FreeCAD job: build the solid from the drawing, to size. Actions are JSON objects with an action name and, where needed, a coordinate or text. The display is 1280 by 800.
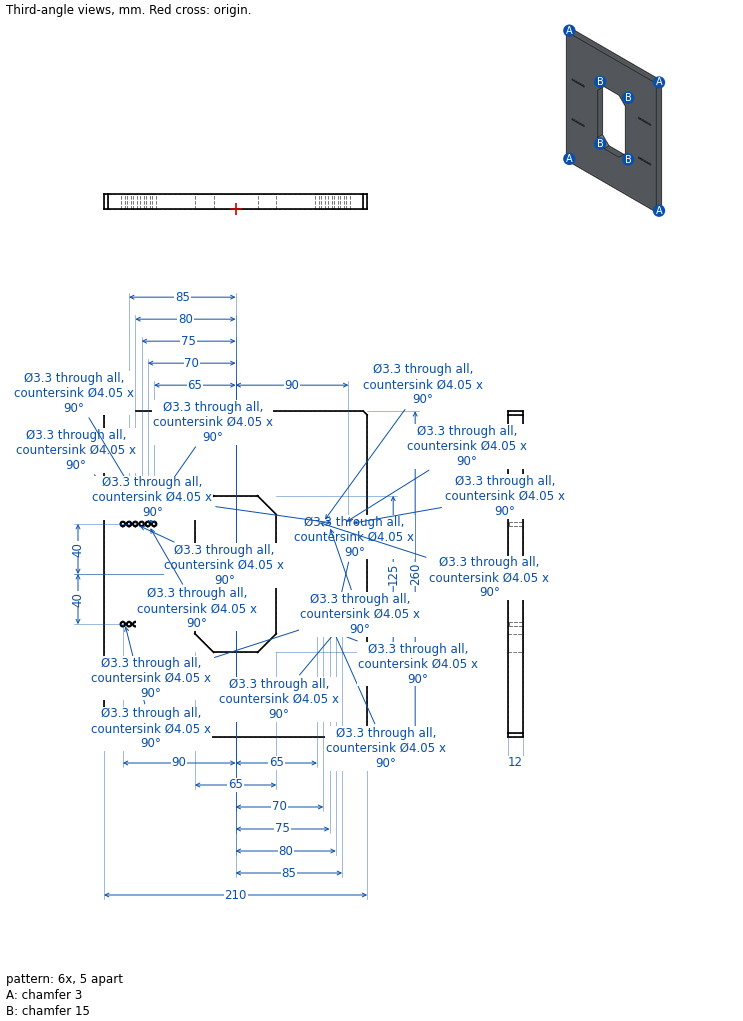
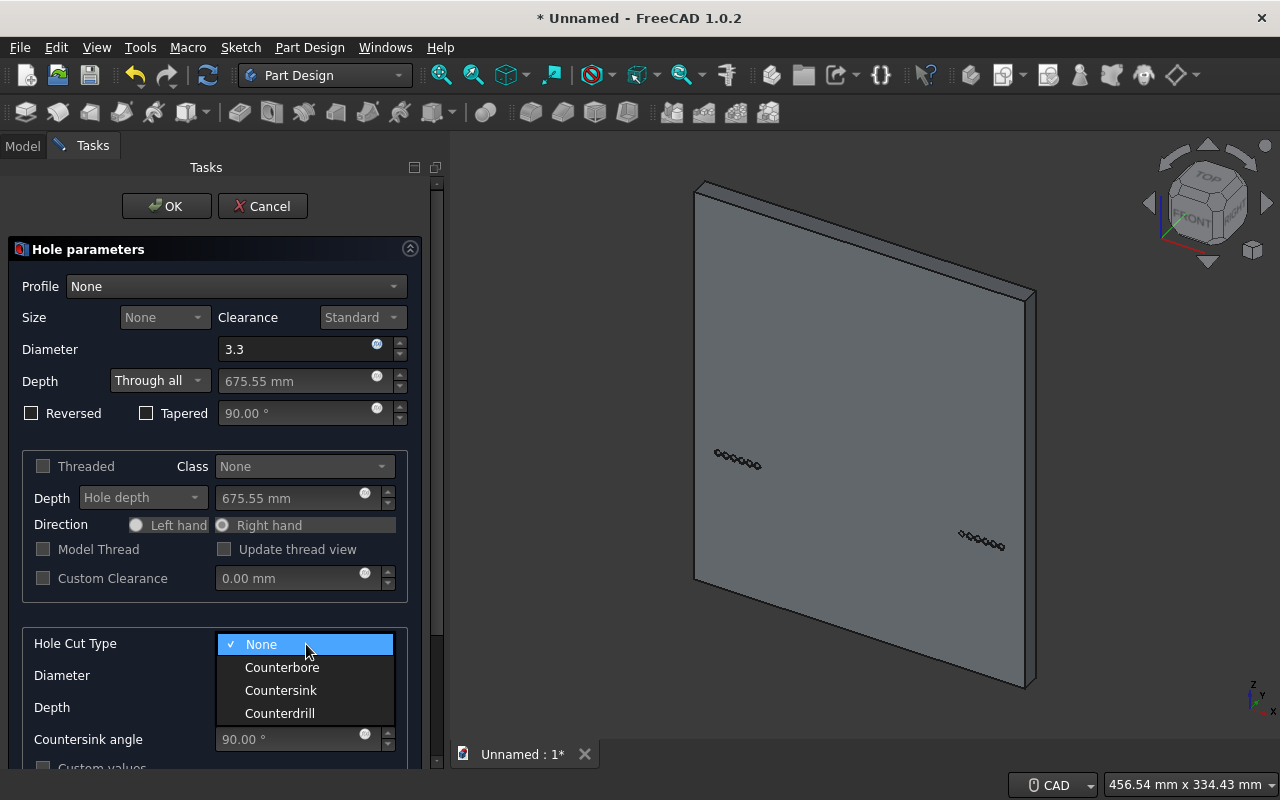
{"action": "left_click", "coordinate": [304, 690]}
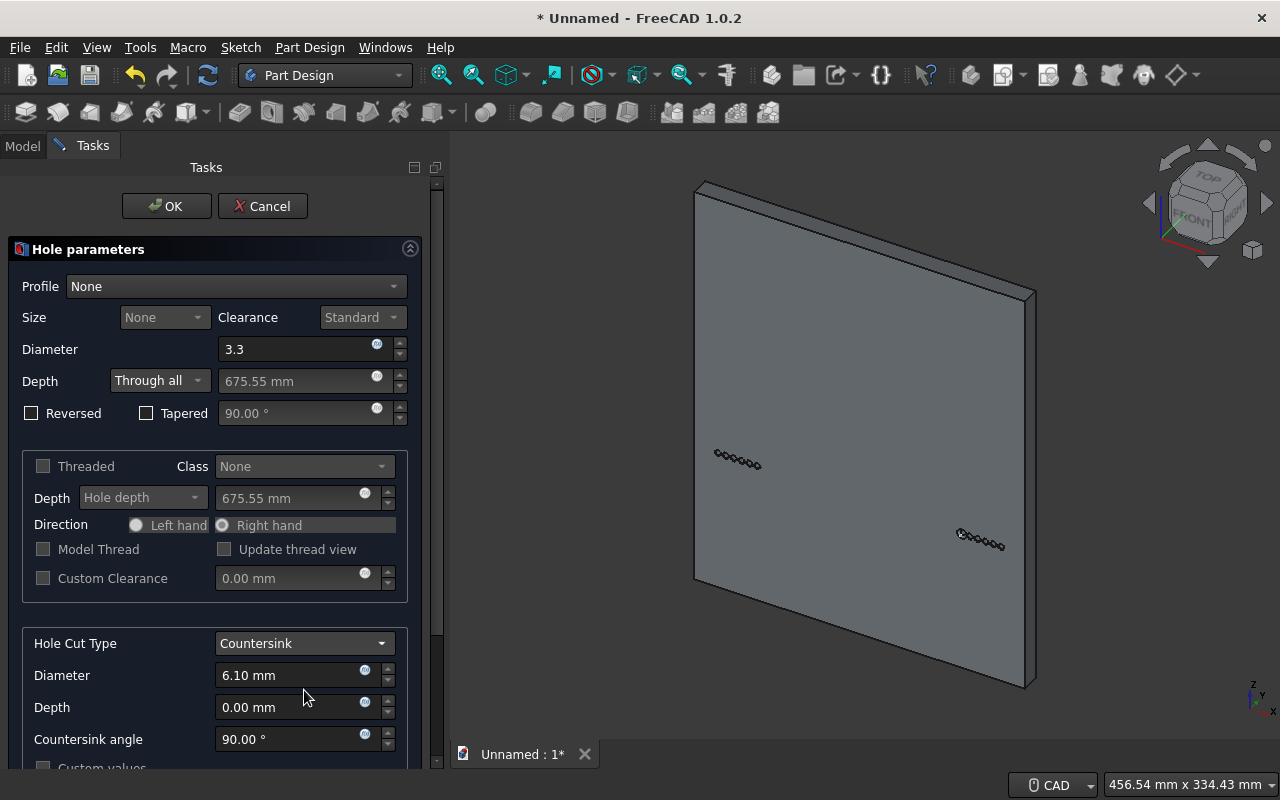
{"action": "triple_click", "coordinate": [298, 675]}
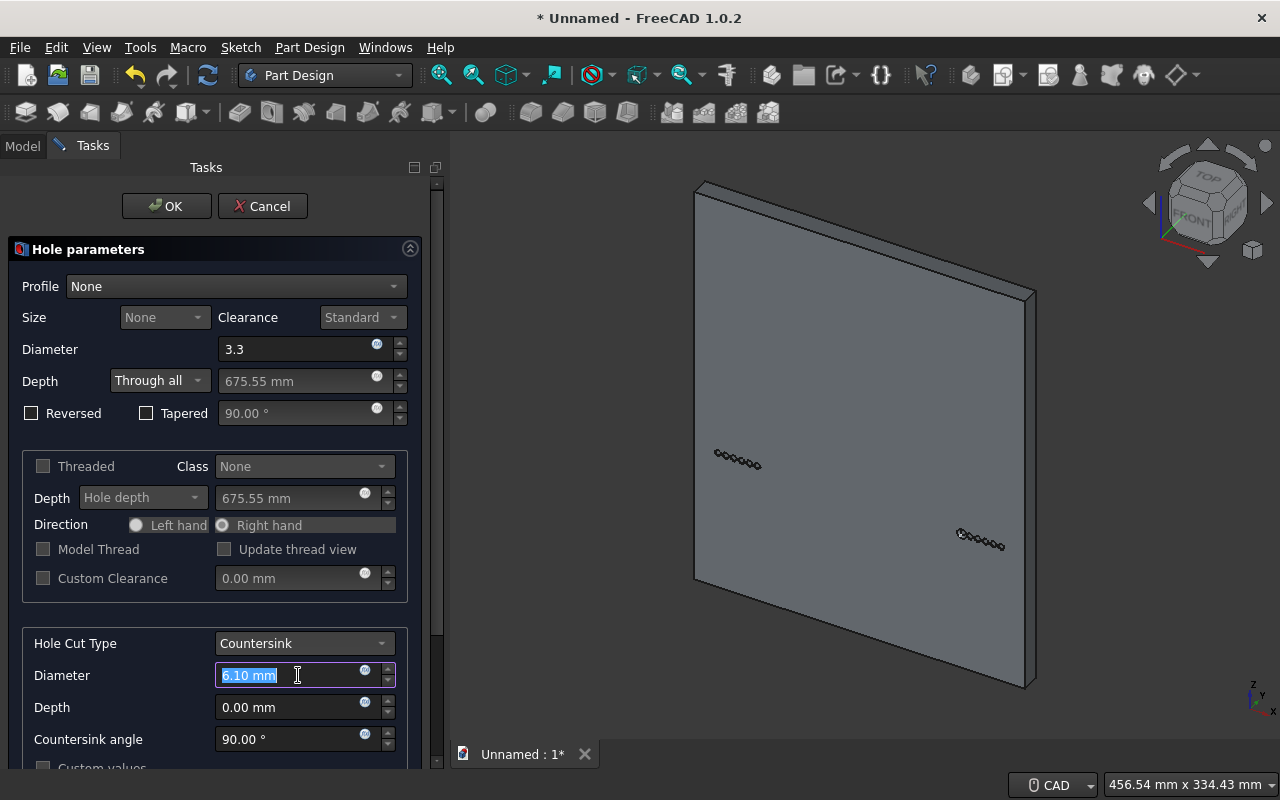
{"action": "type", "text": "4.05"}
{"action": "key", "text": "Tab"}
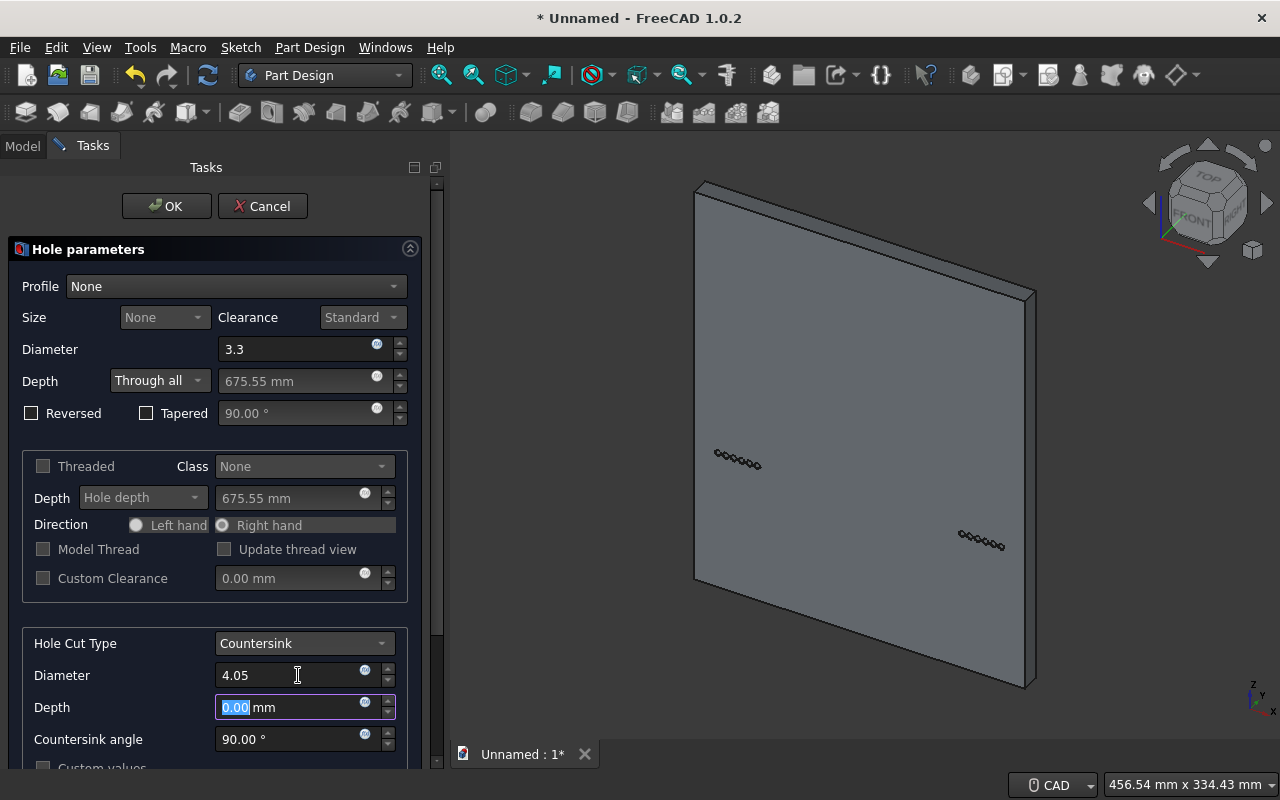
{"action": "left_click", "coordinate": [167, 206]}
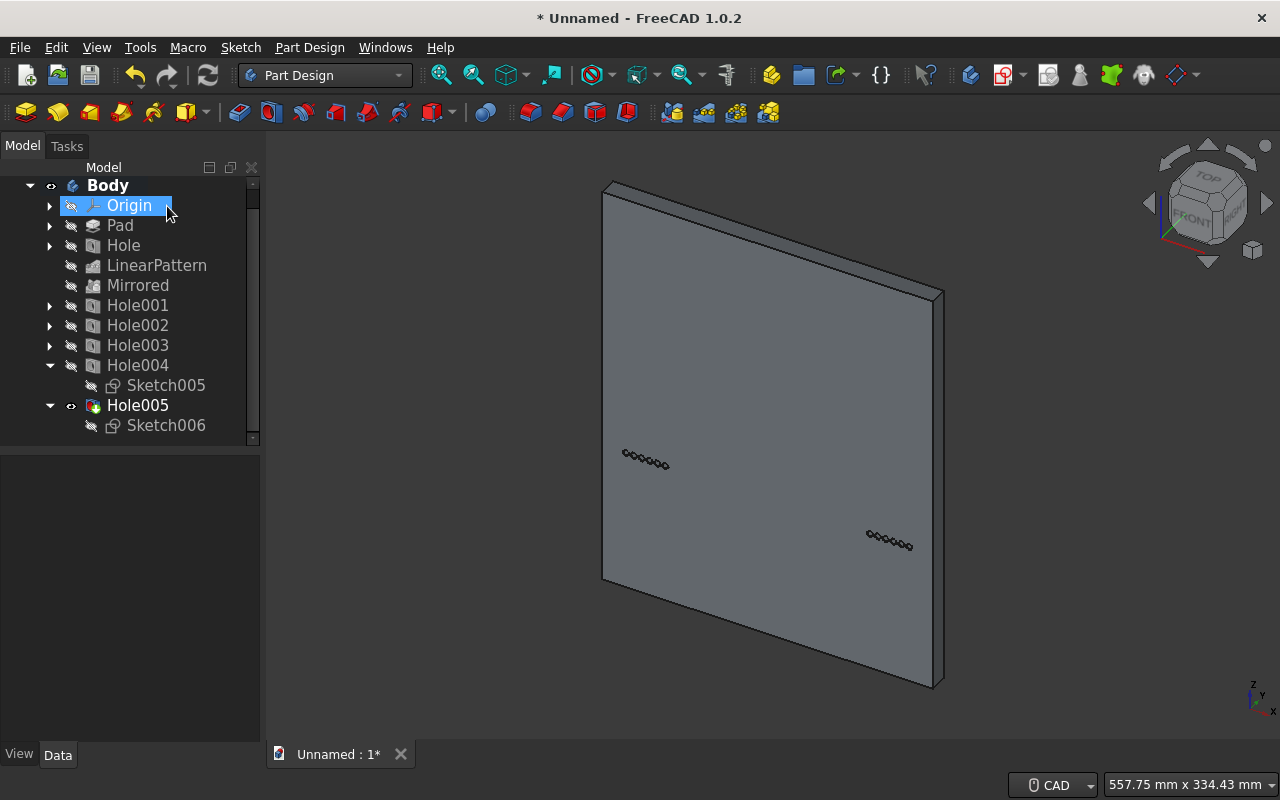
{"action": "left_click", "coordinate": [116, 246]}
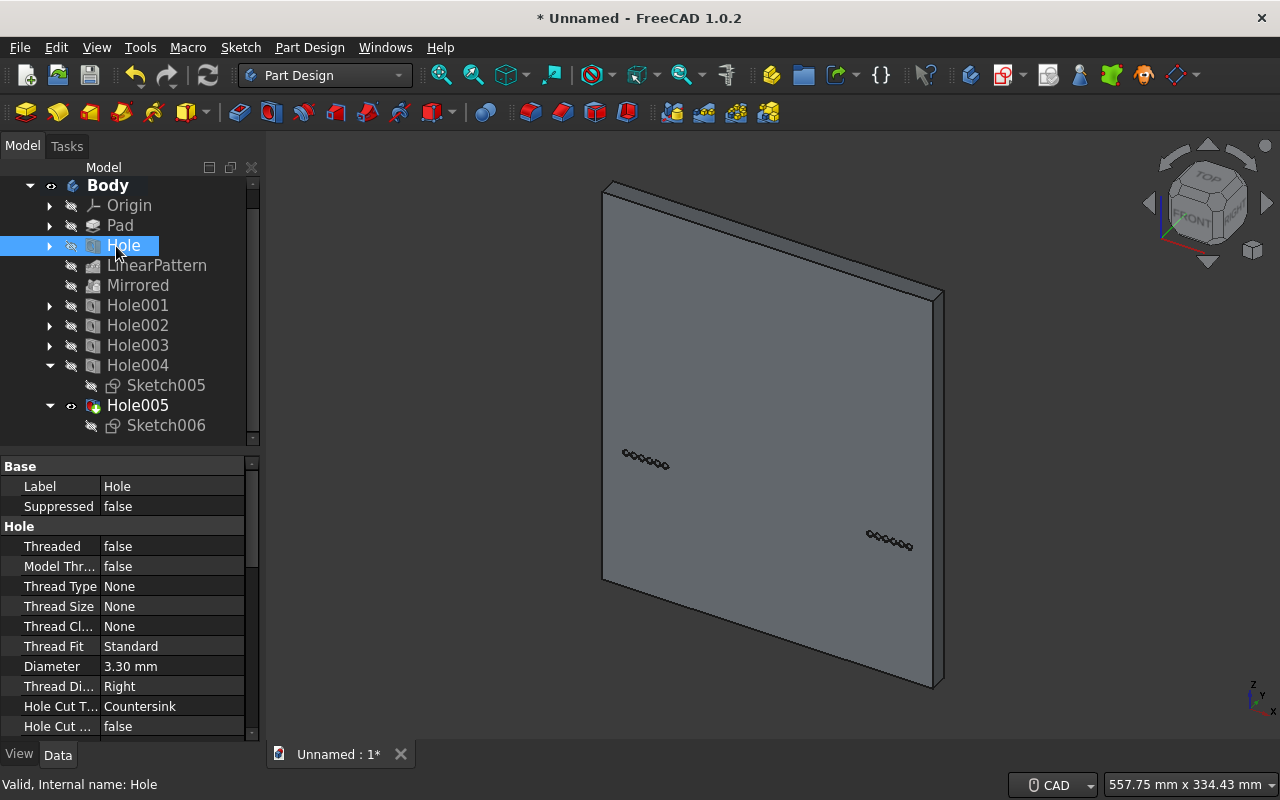
{"action": "left_click", "coordinate": [672, 112]}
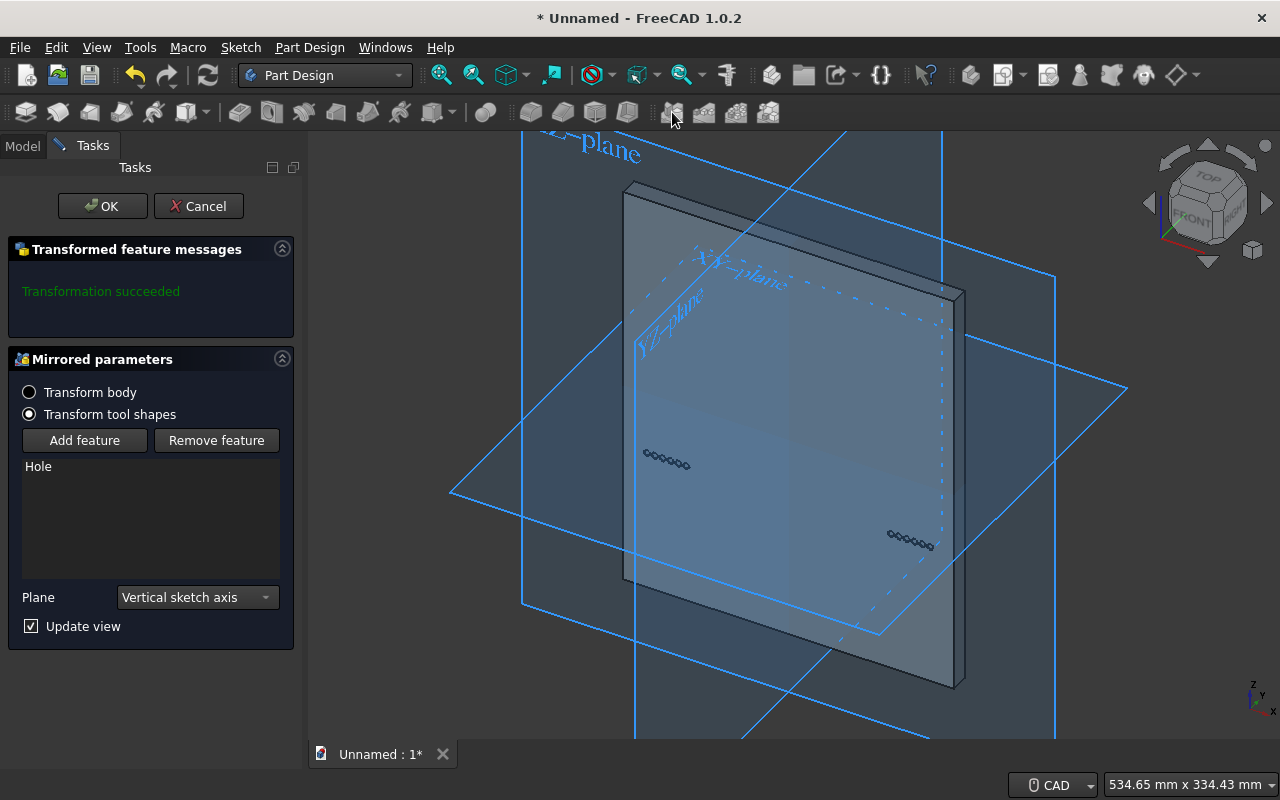
{"action": "left_click", "coordinate": [198, 598]}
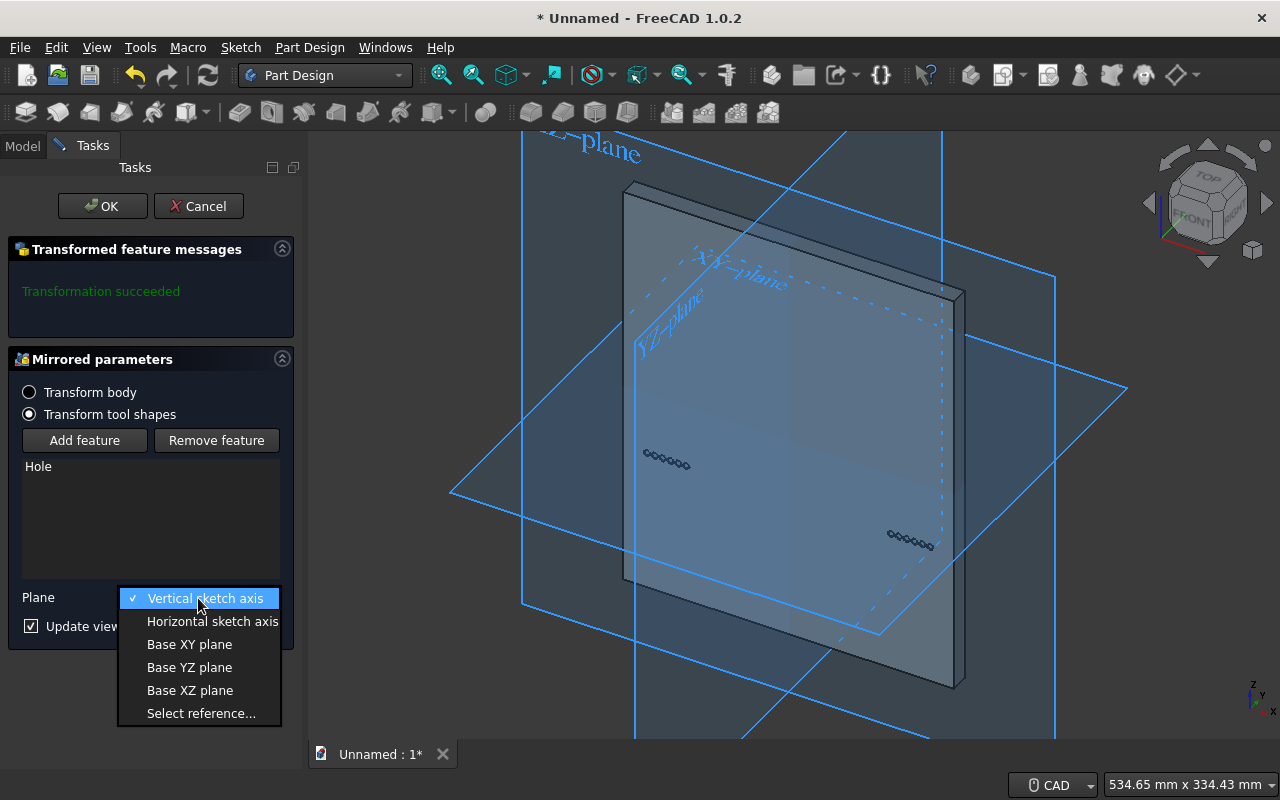
{"action": "left_click", "coordinate": [198, 644]}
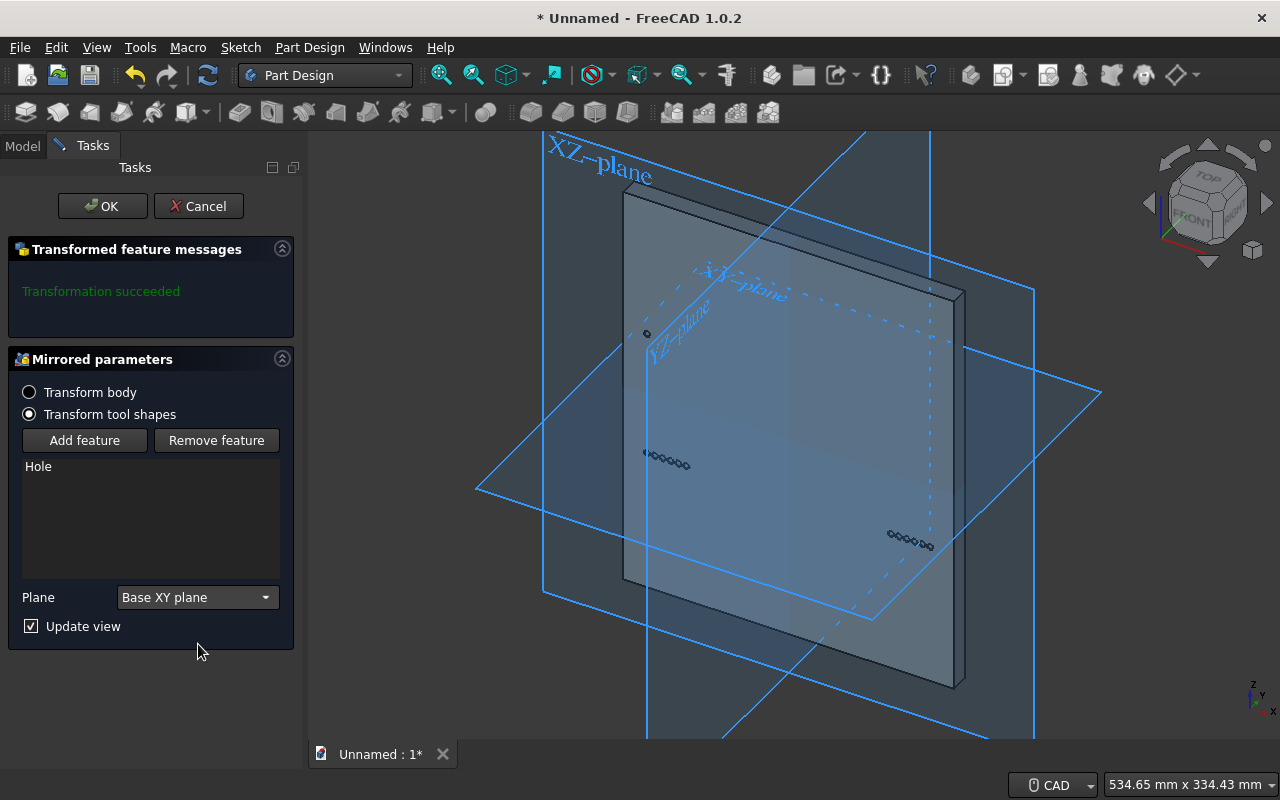
{"action": "left_click", "coordinate": [103, 206]}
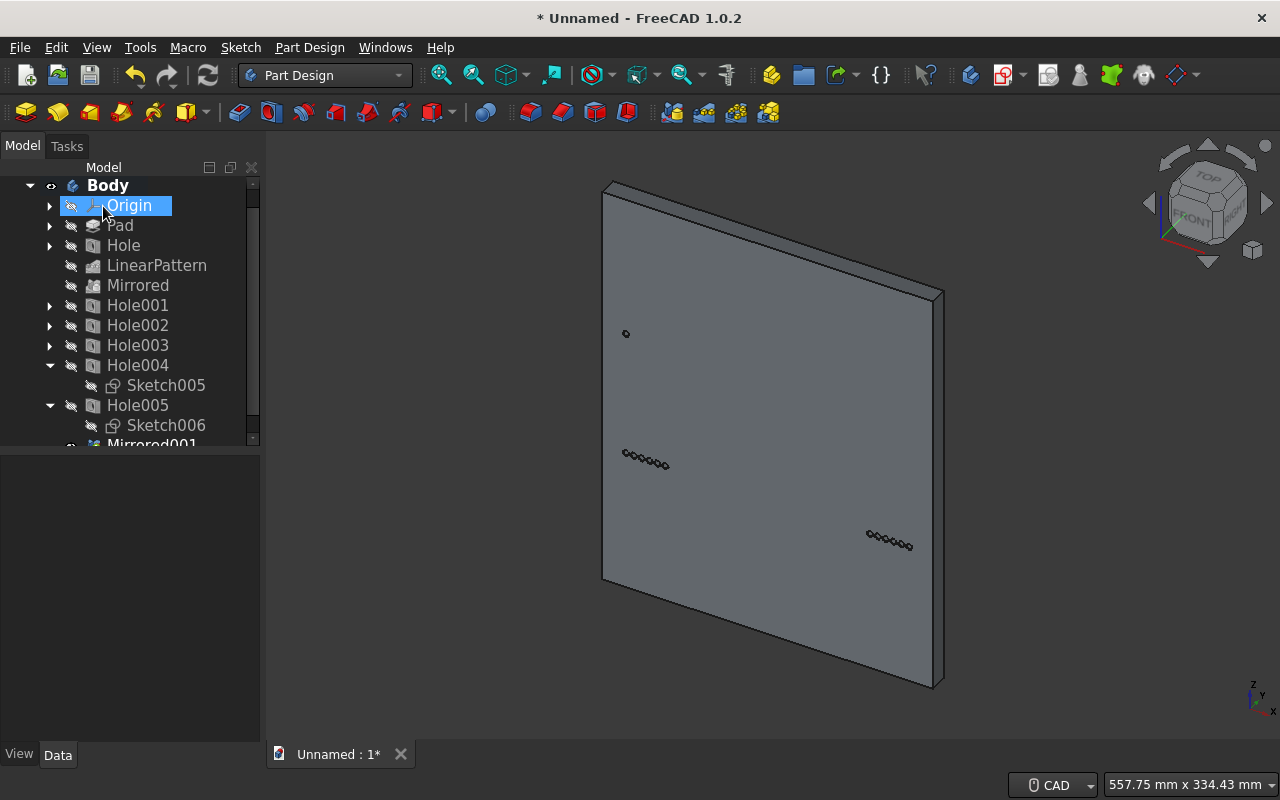
{"action": "left_click", "coordinate": [768, 384]}